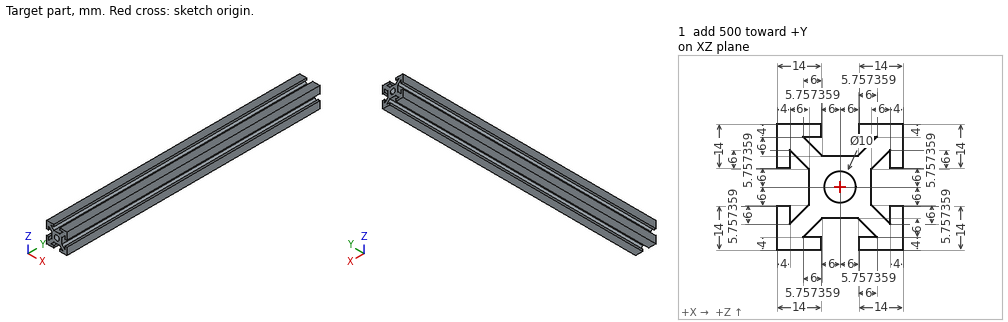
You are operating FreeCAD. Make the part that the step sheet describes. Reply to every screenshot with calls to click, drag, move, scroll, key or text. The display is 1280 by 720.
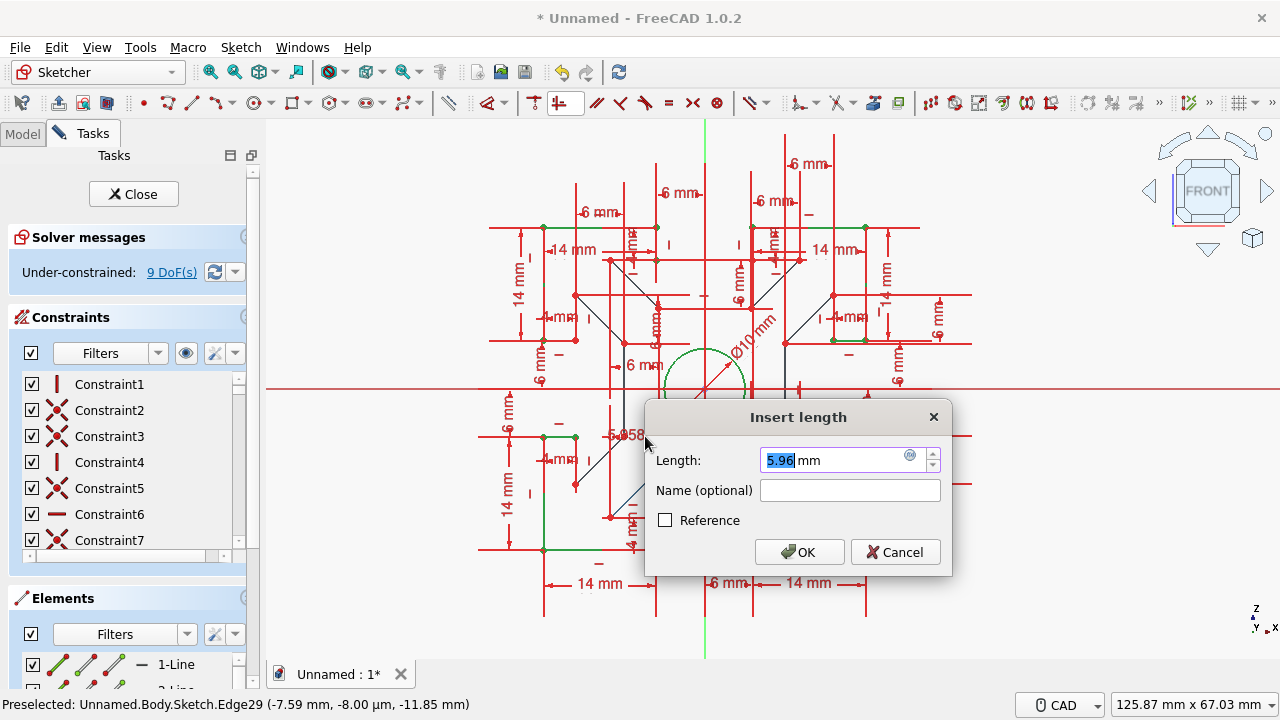
text(6)
key(Return)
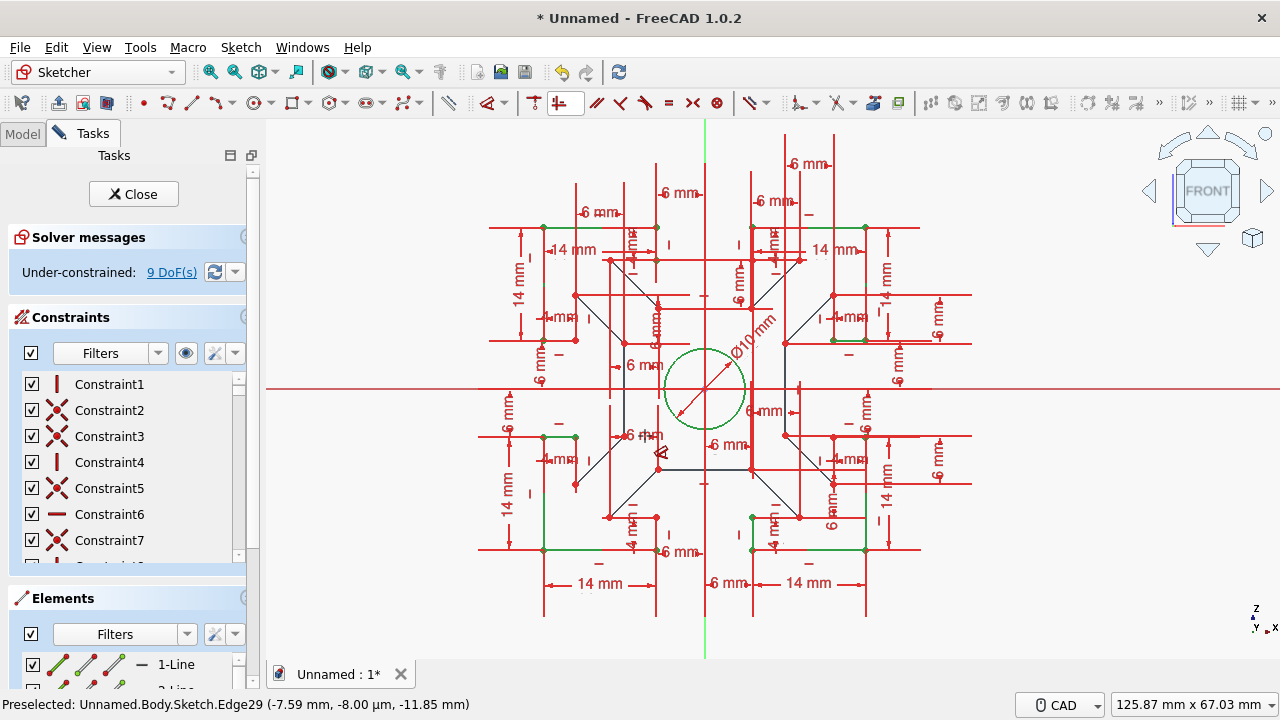
click(590, 470)
click(470, 460)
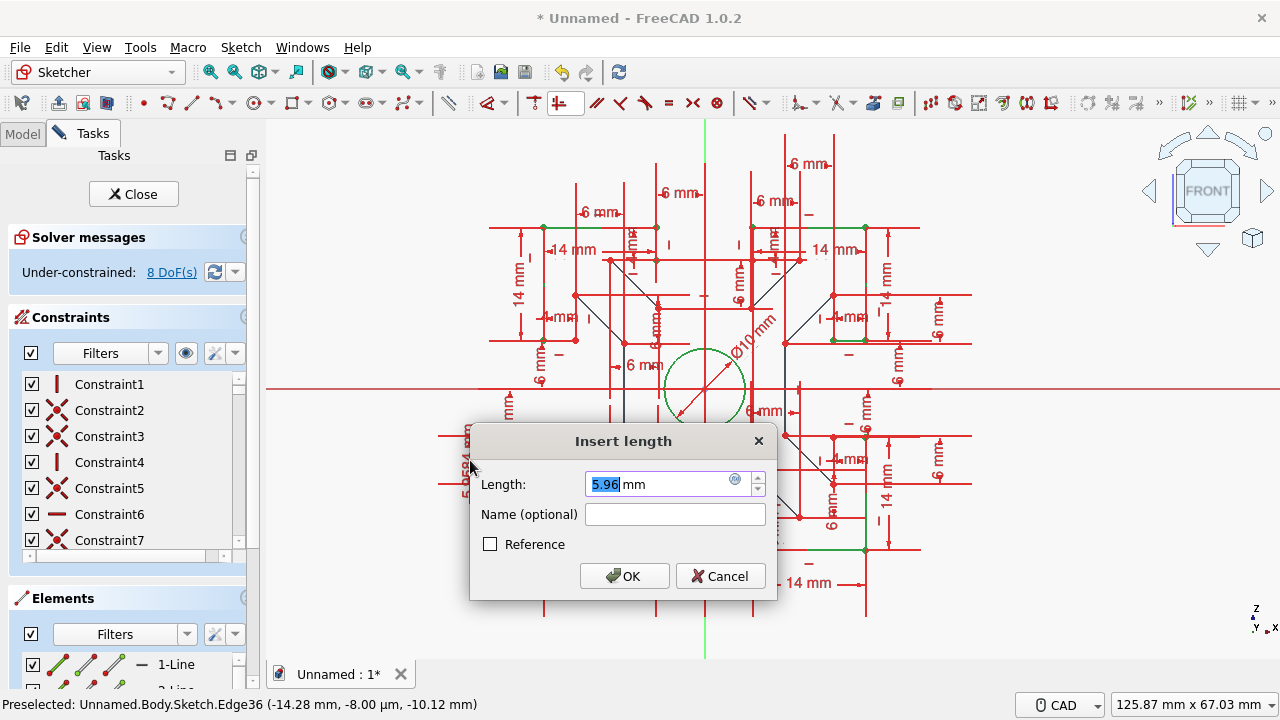
text(6)
key(Return)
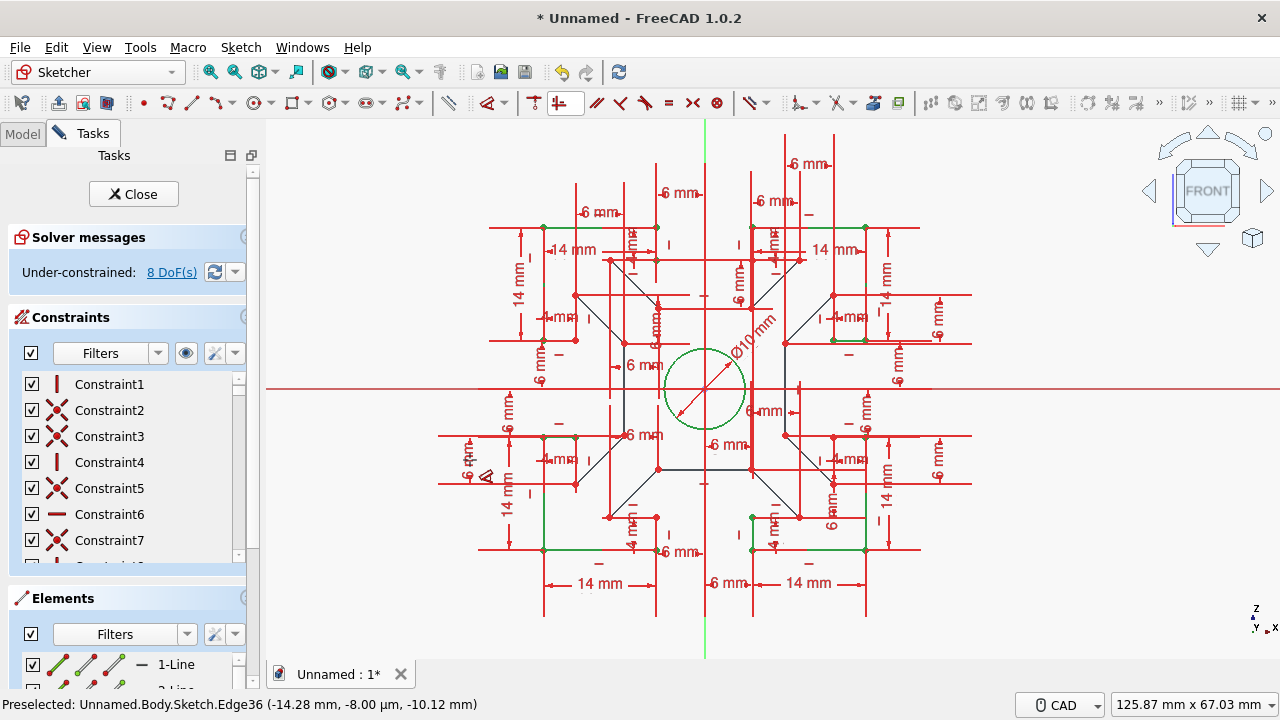
scroll(576, 309, up, 2)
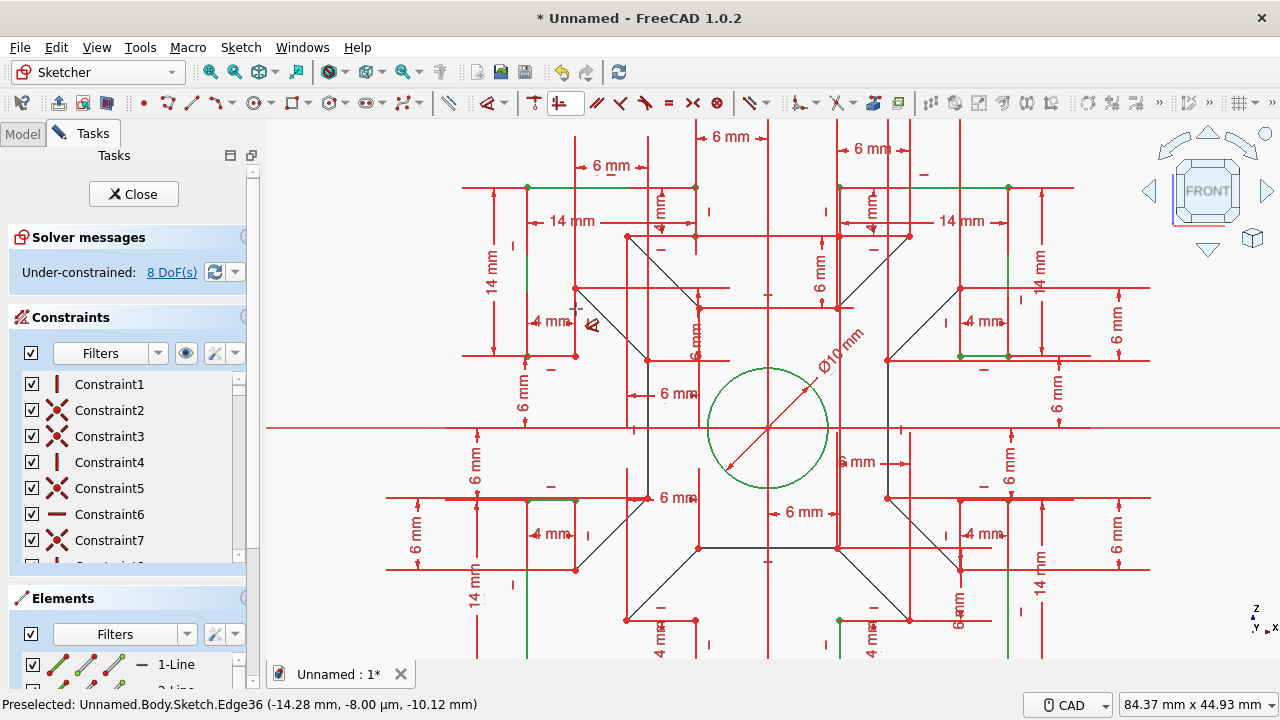
click(575, 309)
click(541, 299)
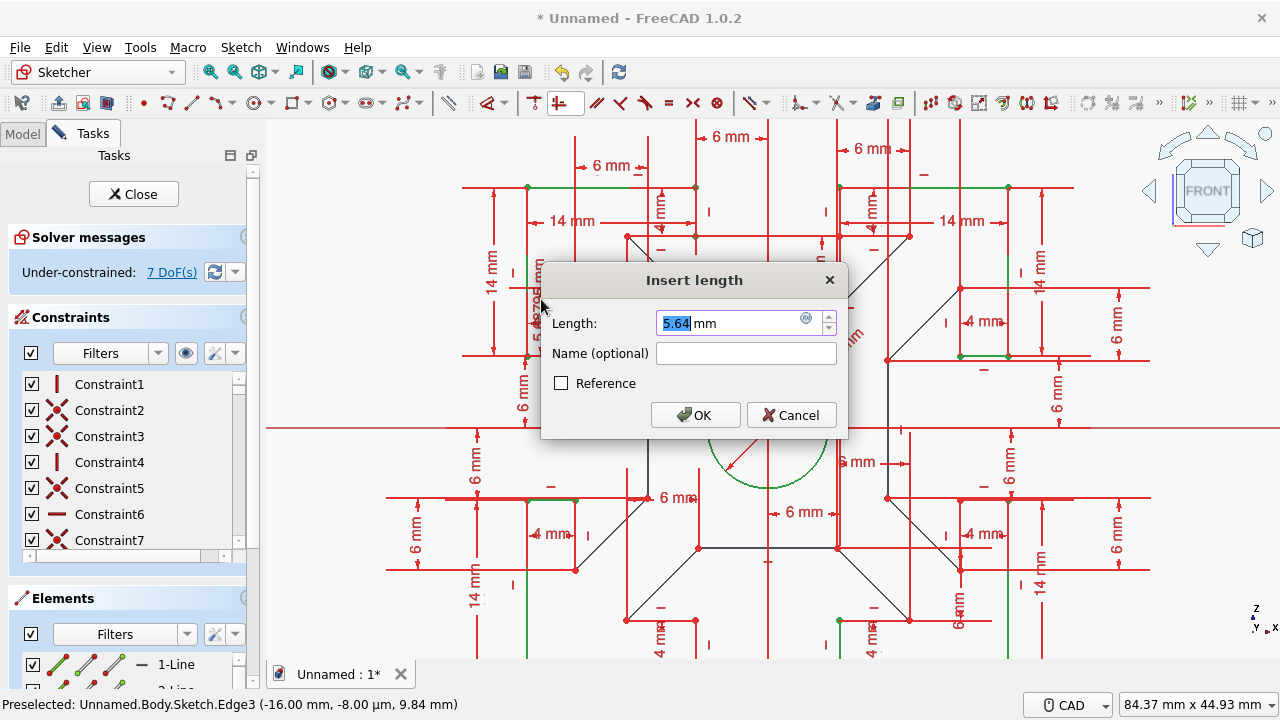
text(5.757359)
key(Return)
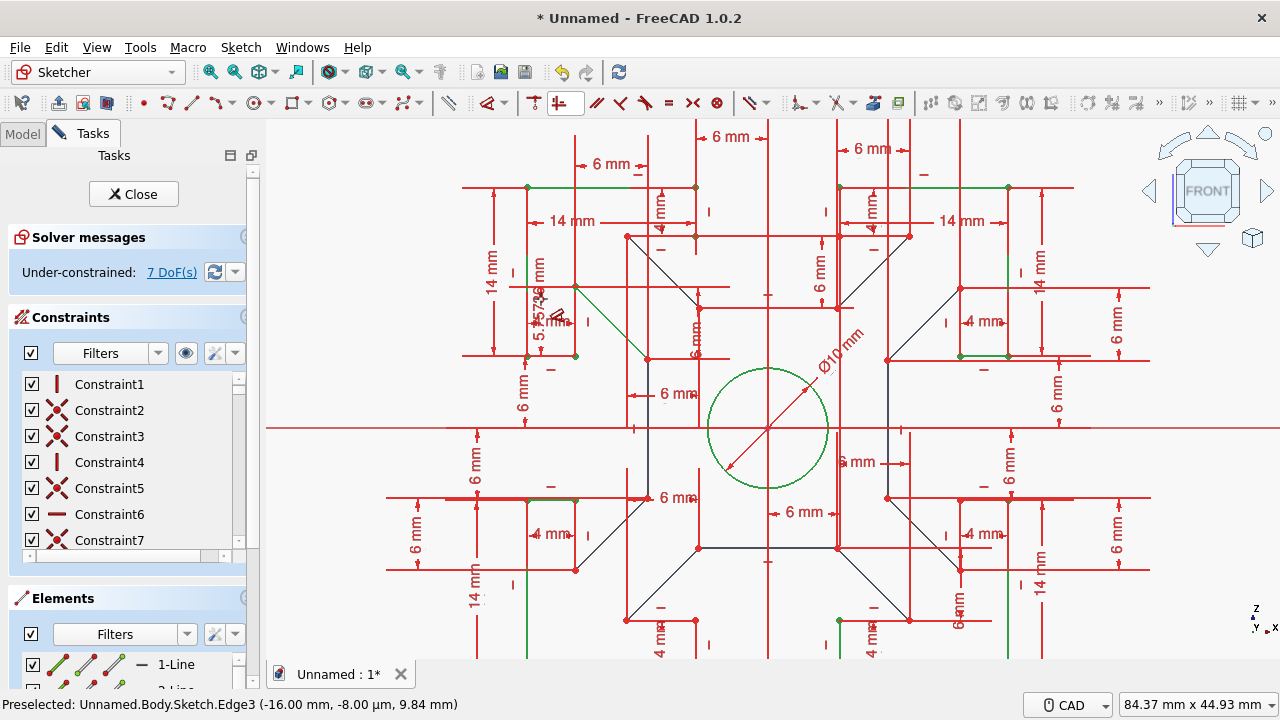
click(675, 236)
click(637, 270)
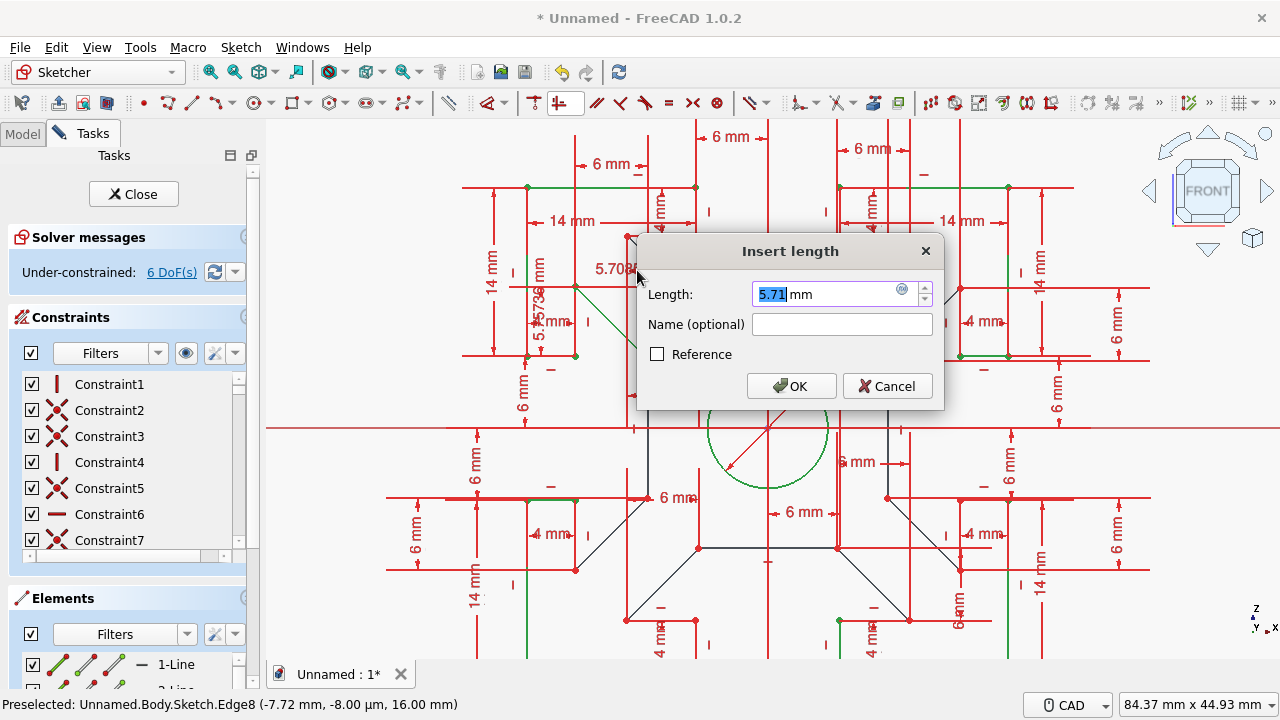
text(5.757359)
key(Return)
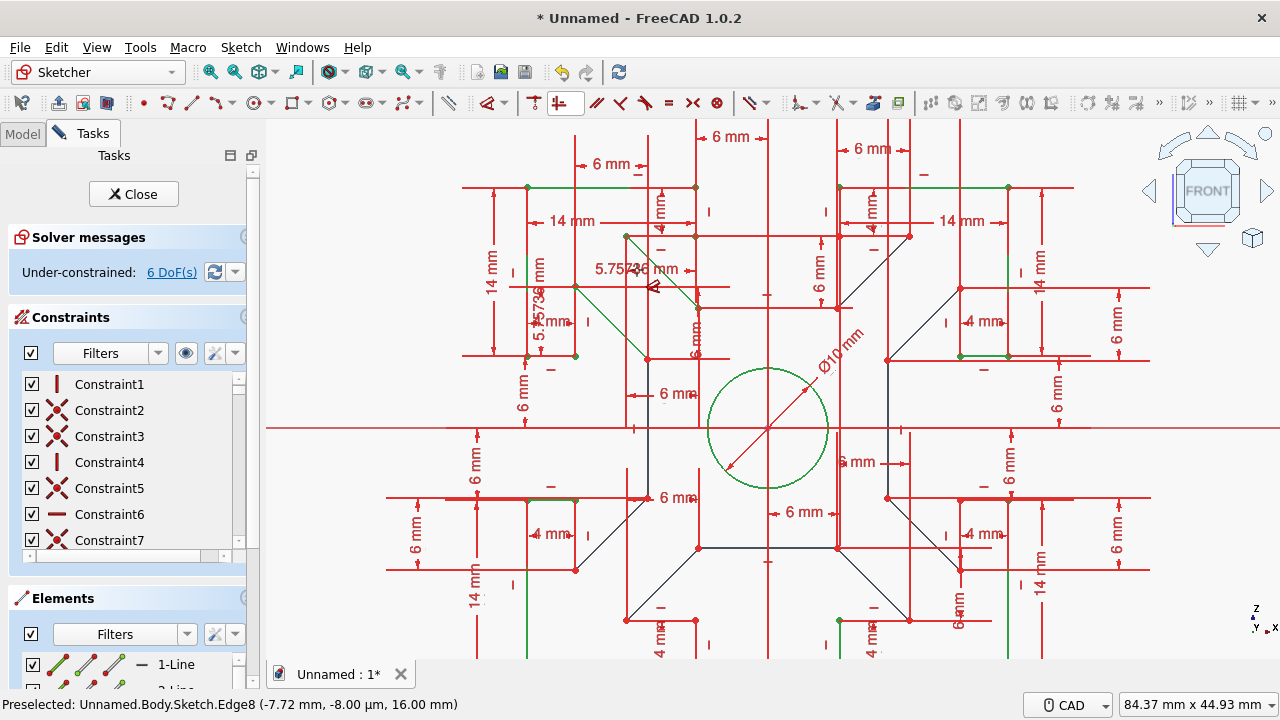
click(889, 236)
click(899, 270)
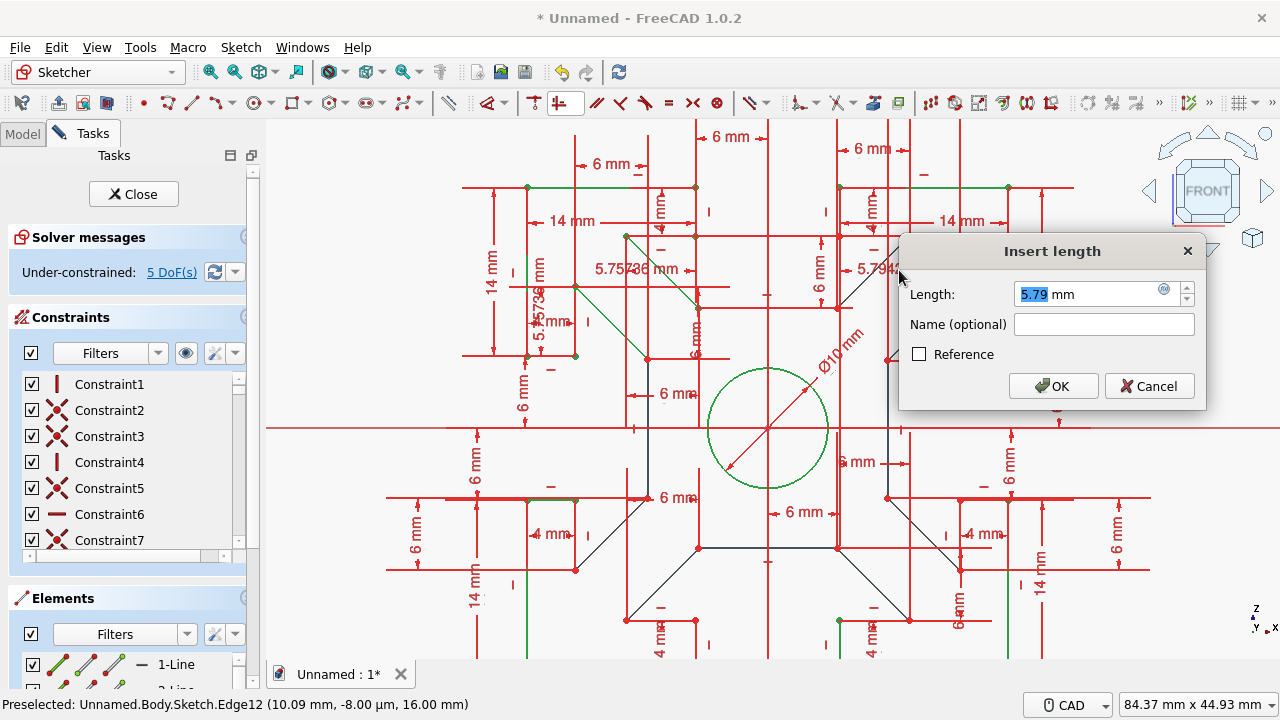
text(5.757359)
key(Return)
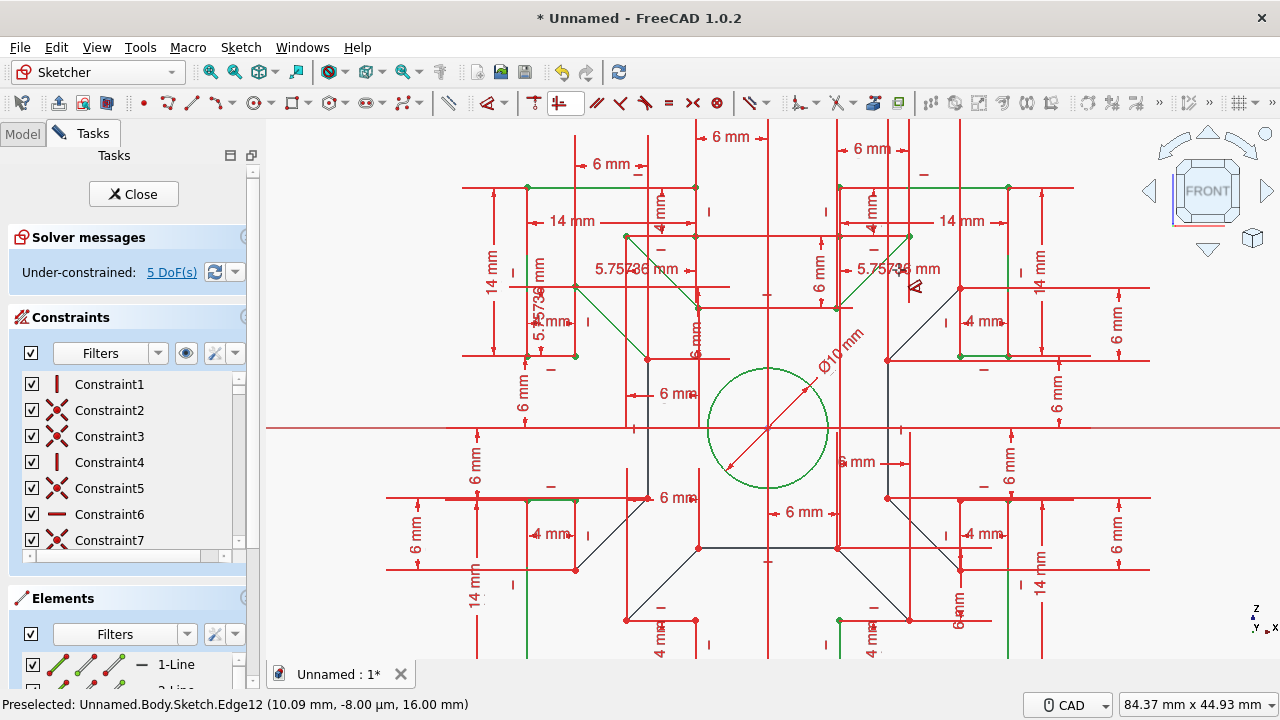
click(960, 336)
click(994, 299)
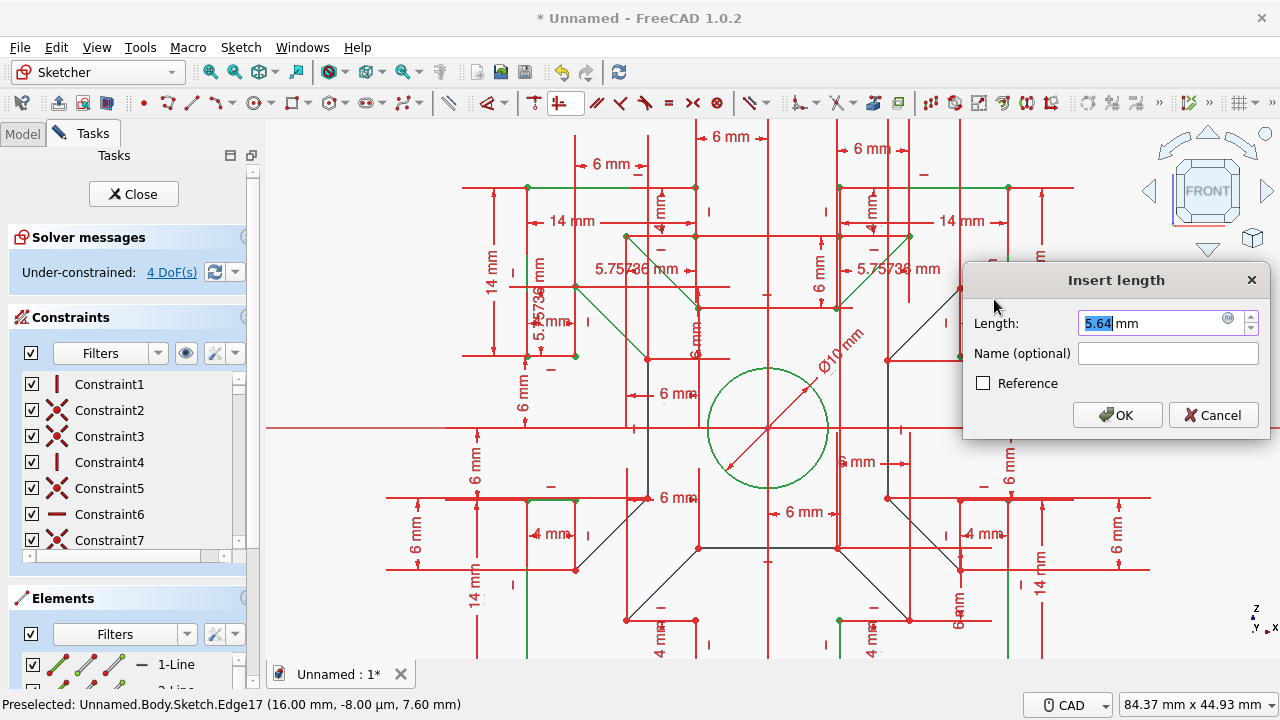
text(5.757359)
key(Return)